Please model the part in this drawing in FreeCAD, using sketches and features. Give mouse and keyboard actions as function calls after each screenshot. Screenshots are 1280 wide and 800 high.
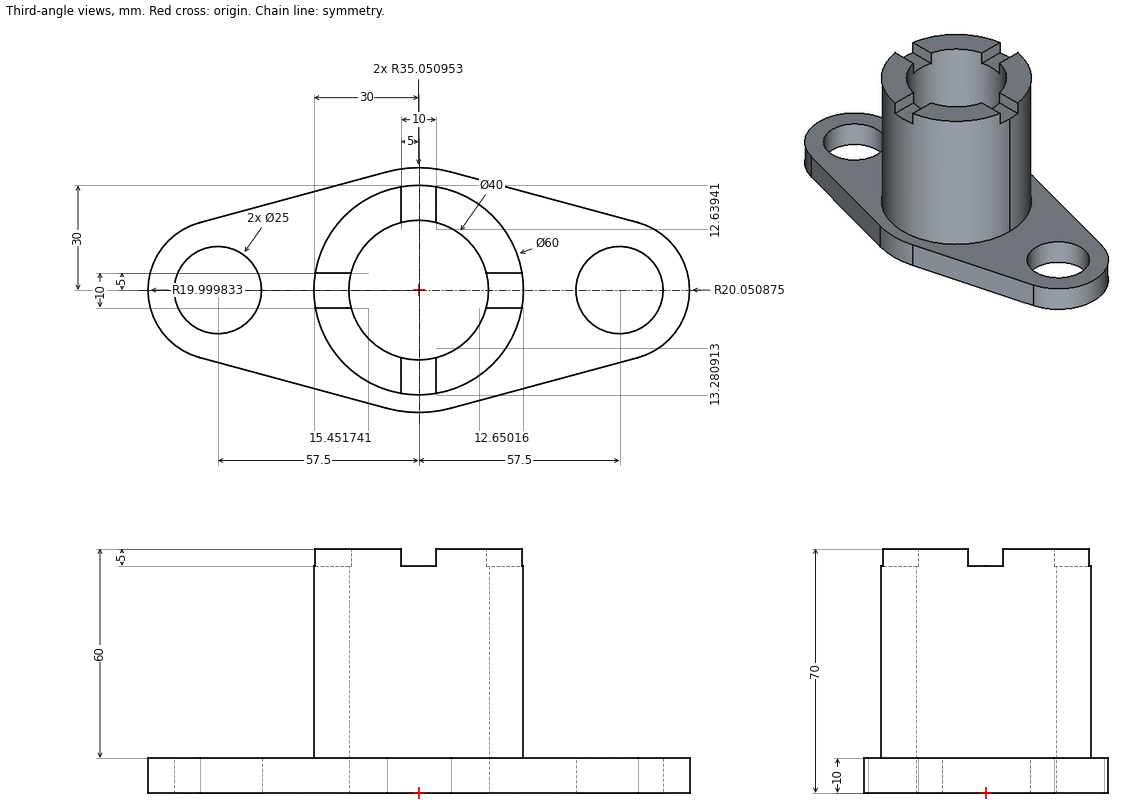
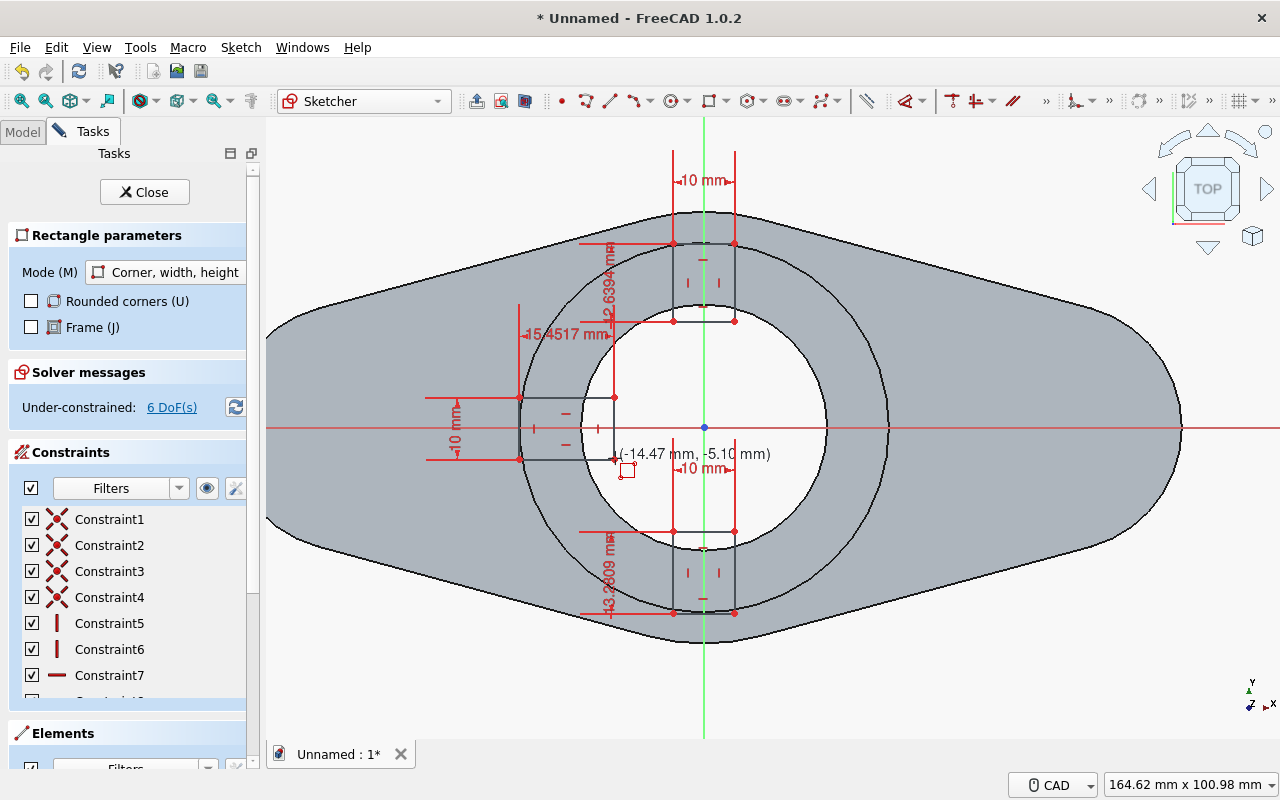
click(811, 397)
move(889, 458)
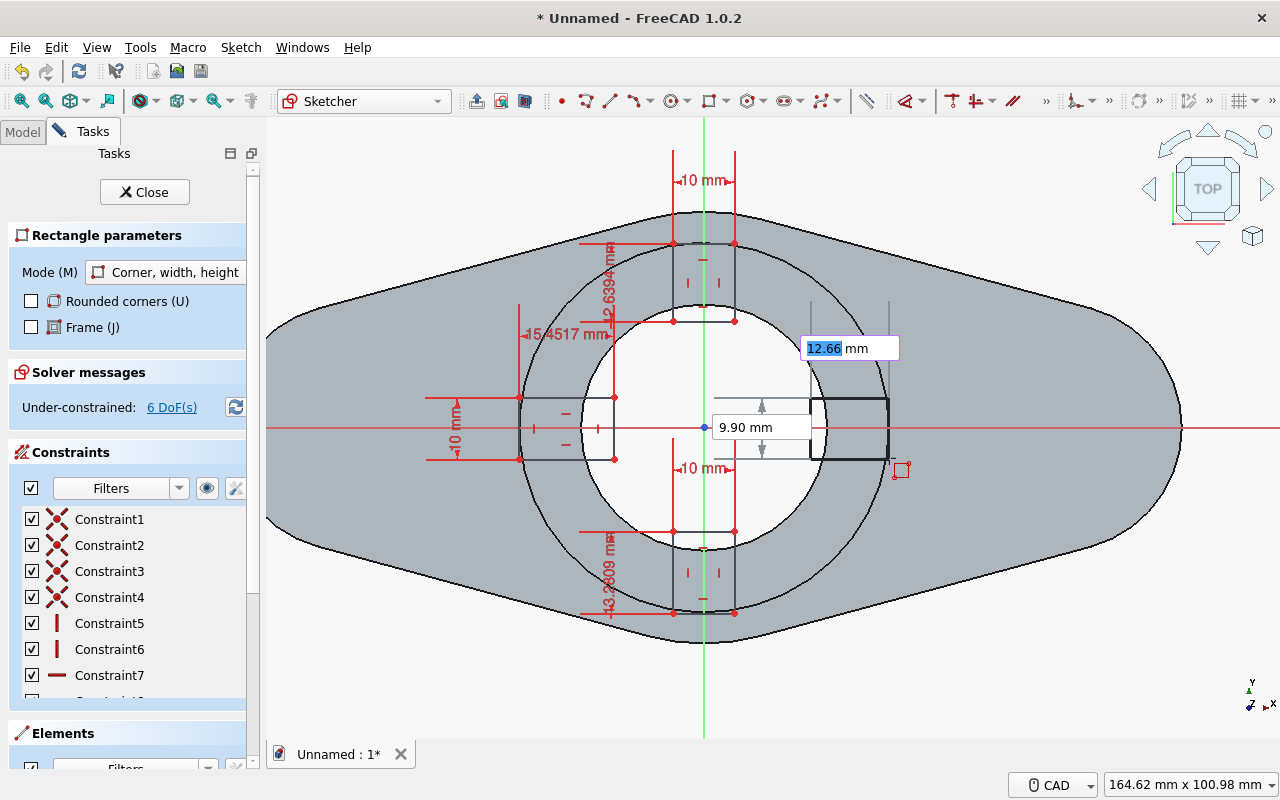
text(12.65016)
key(Tab)
text(10)
key(Return)
key(Escape)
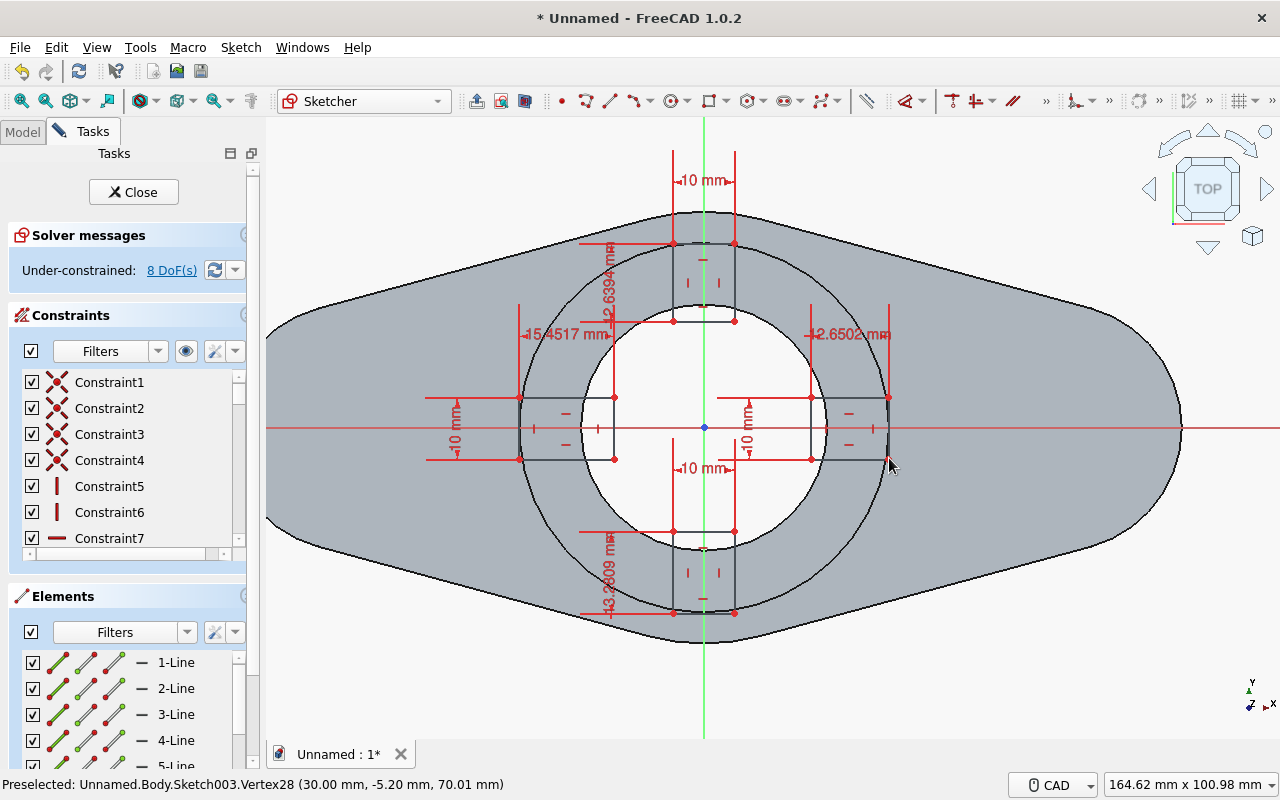
click(673, 244)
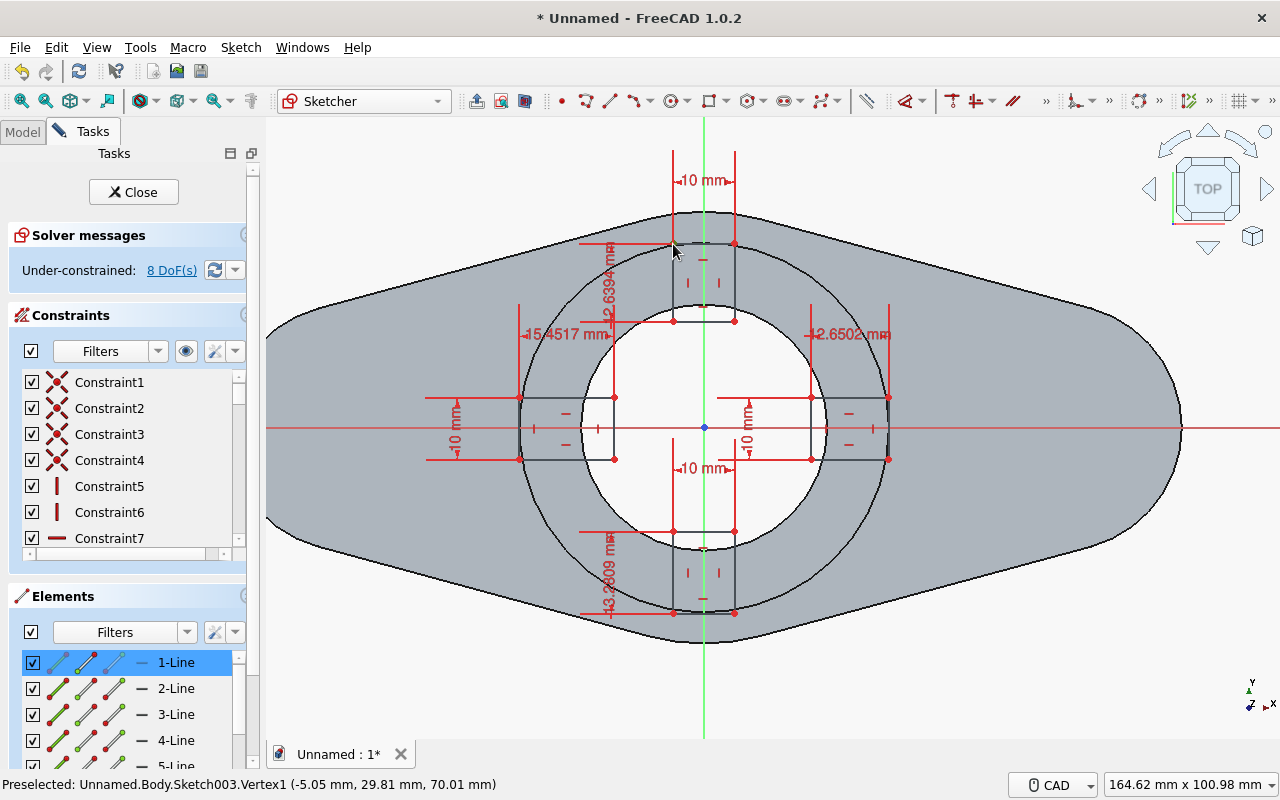
click(673, 614)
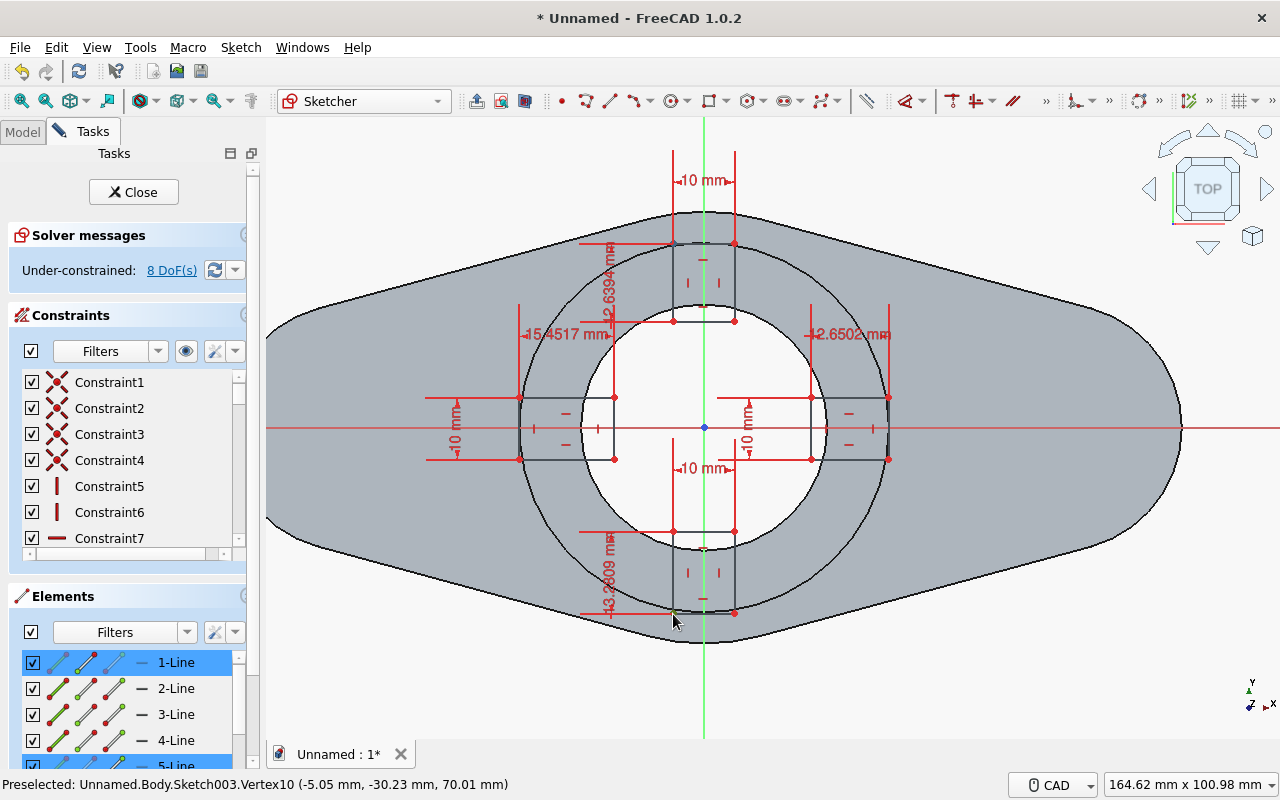
click(353, 428)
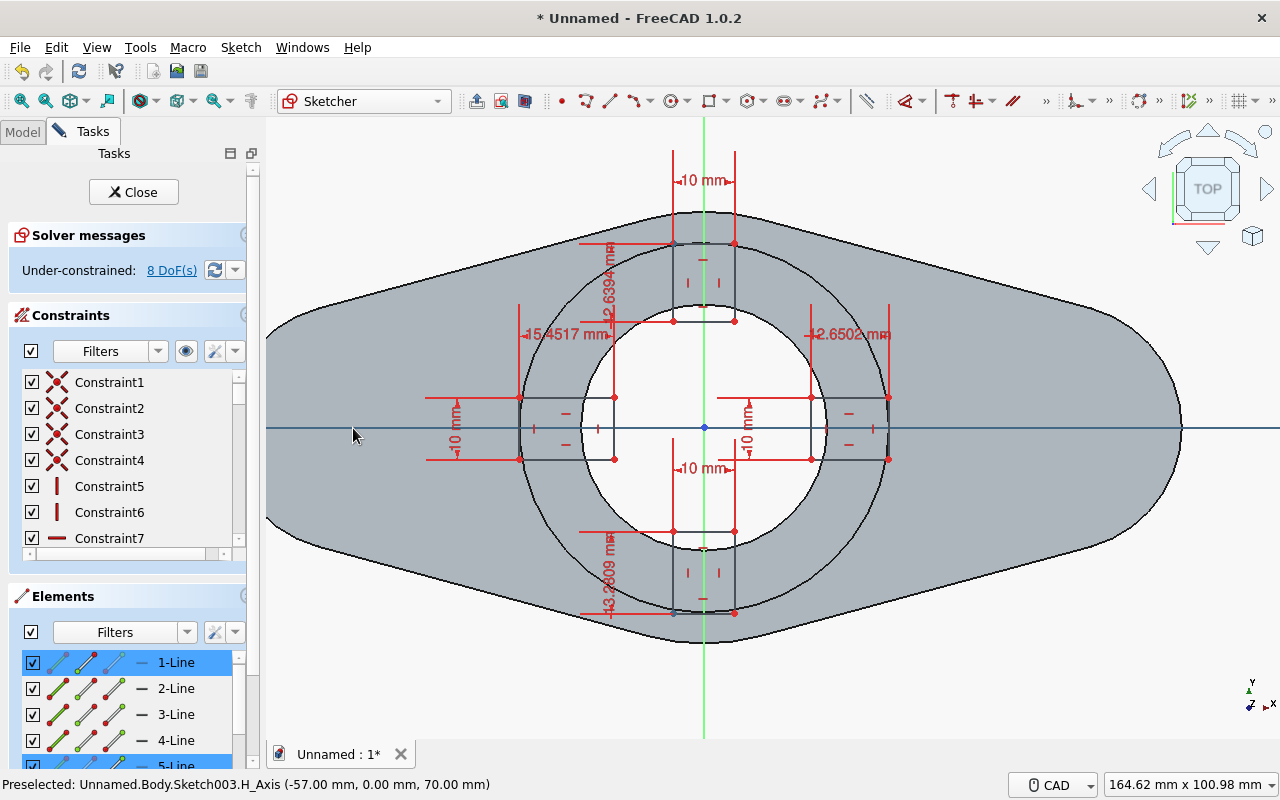
key(s)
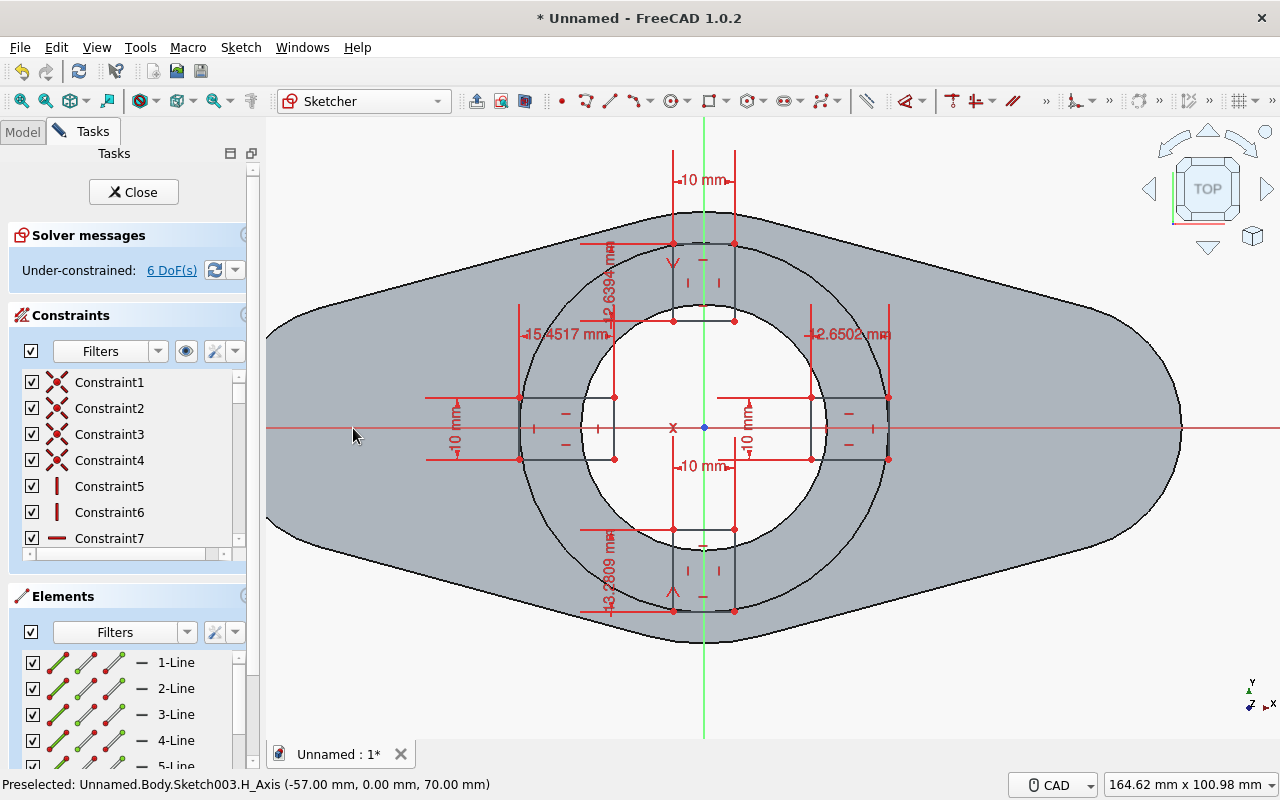
click(519, 460)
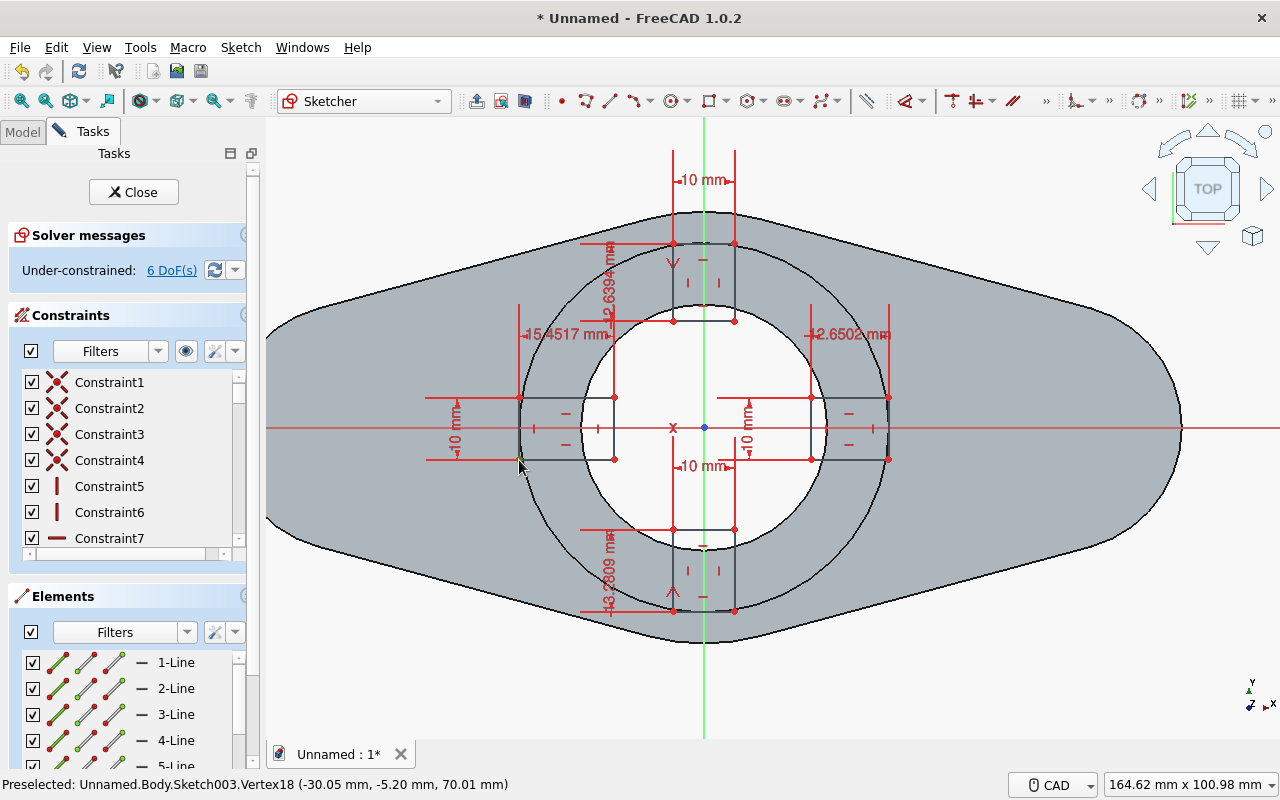
click(889, 460)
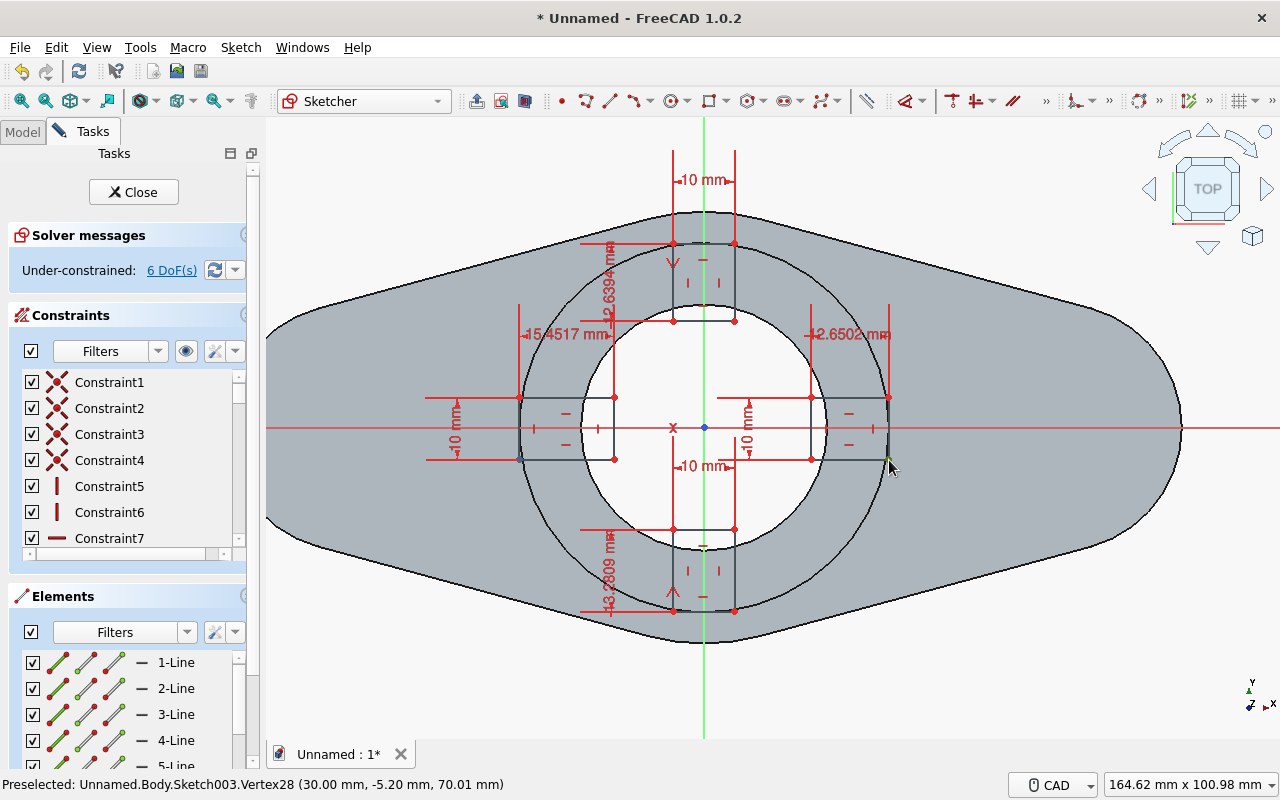
click(704, 671)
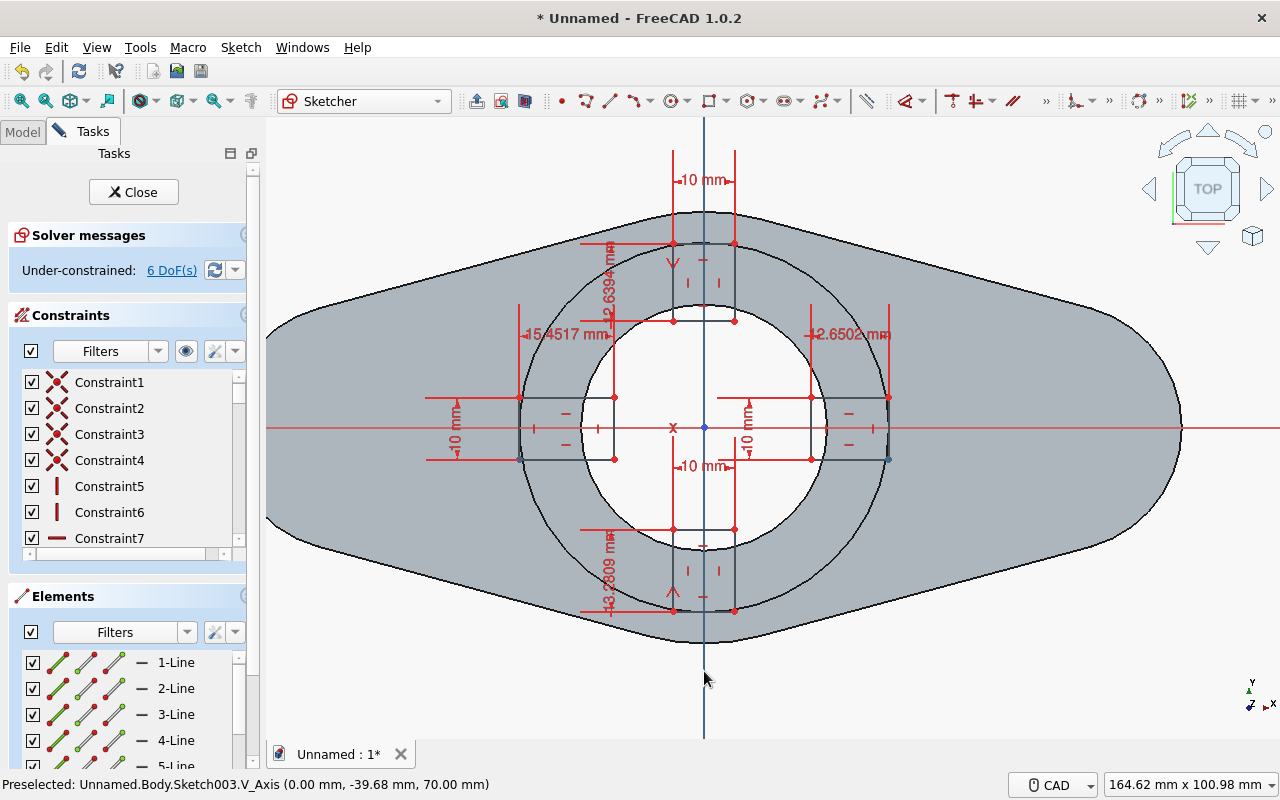
key(s)